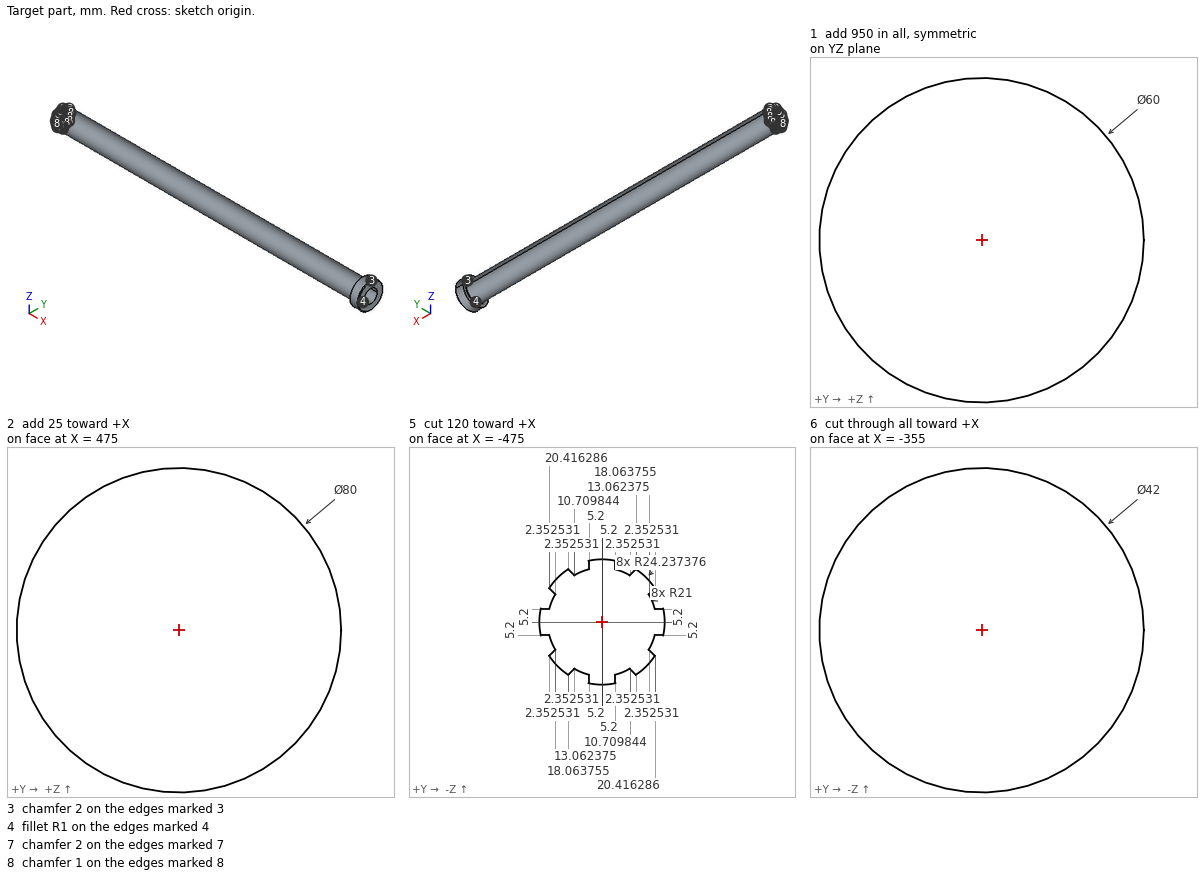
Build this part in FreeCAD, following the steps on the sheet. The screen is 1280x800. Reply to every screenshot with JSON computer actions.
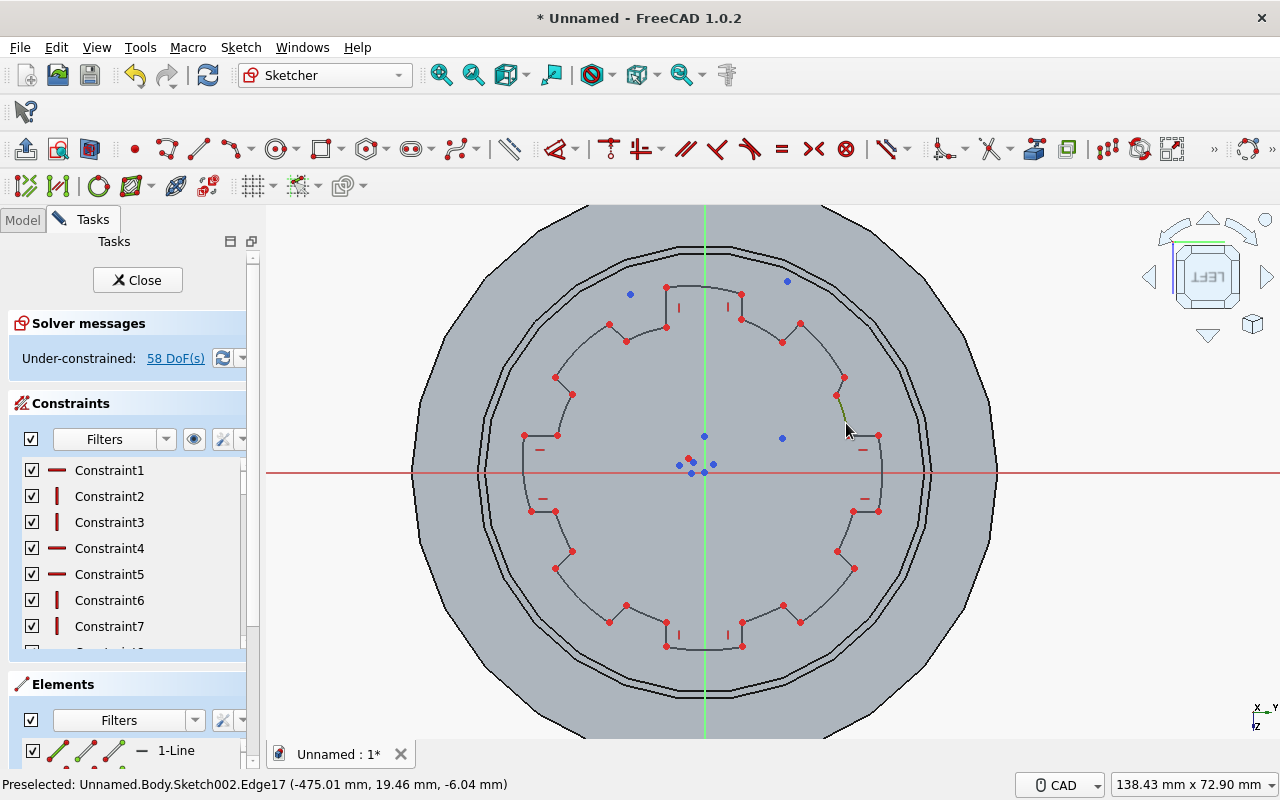
{"action": "left_click", "coordinate": [560, 524]}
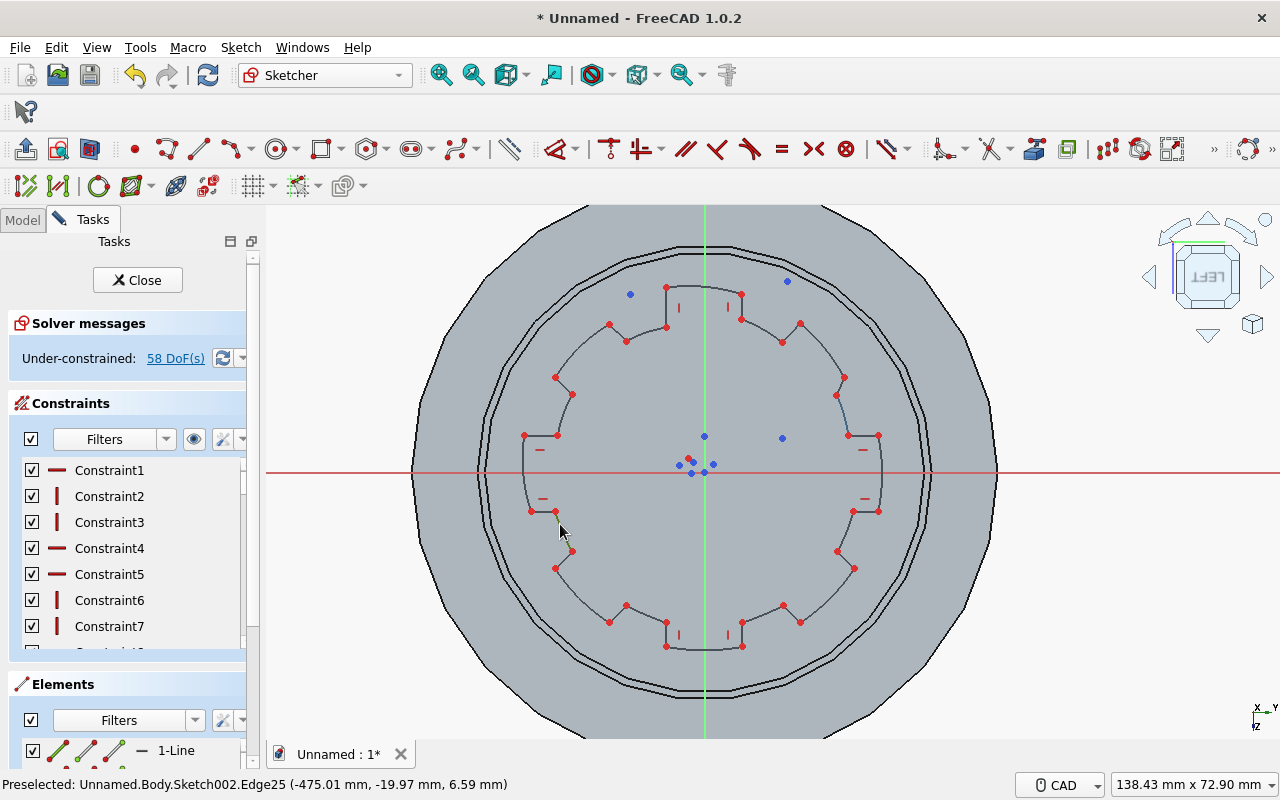
{"action": "key", "text": "c"}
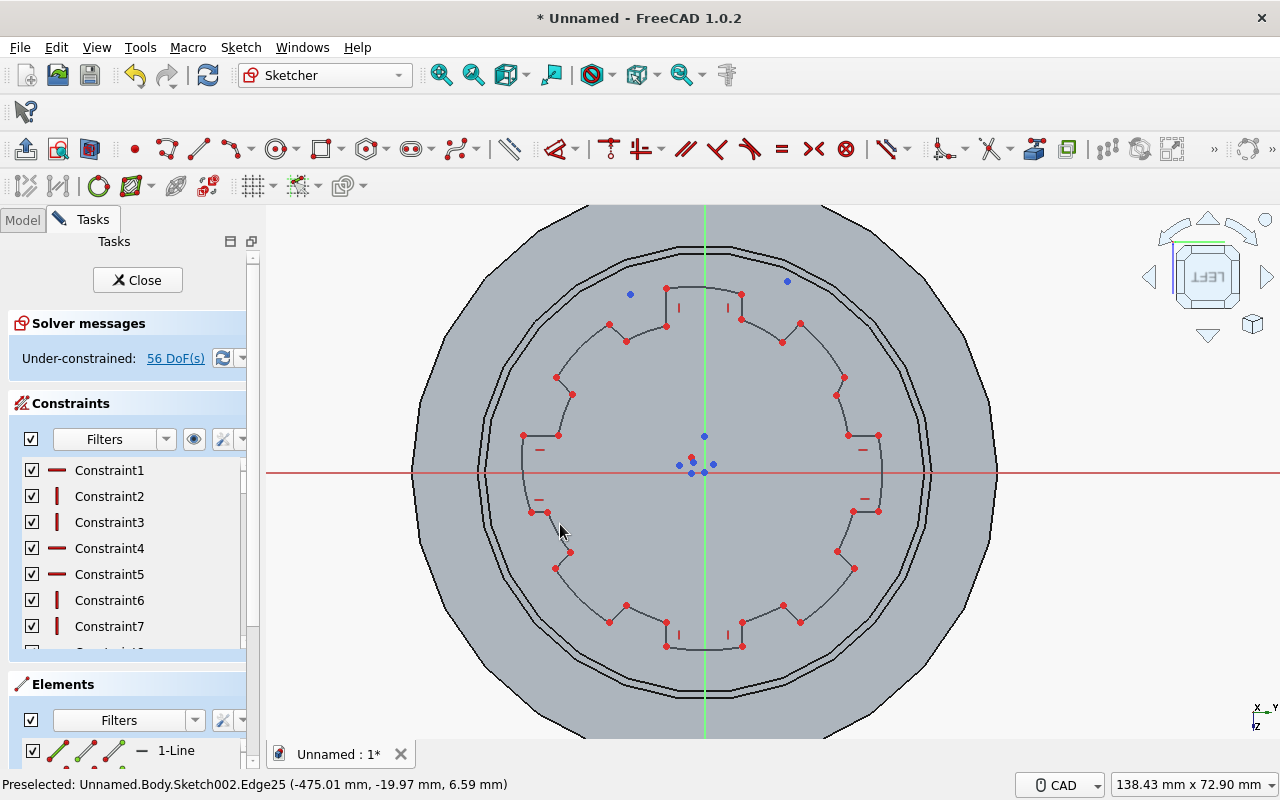
{"action": "left_click", "coordinate": [846, 423]}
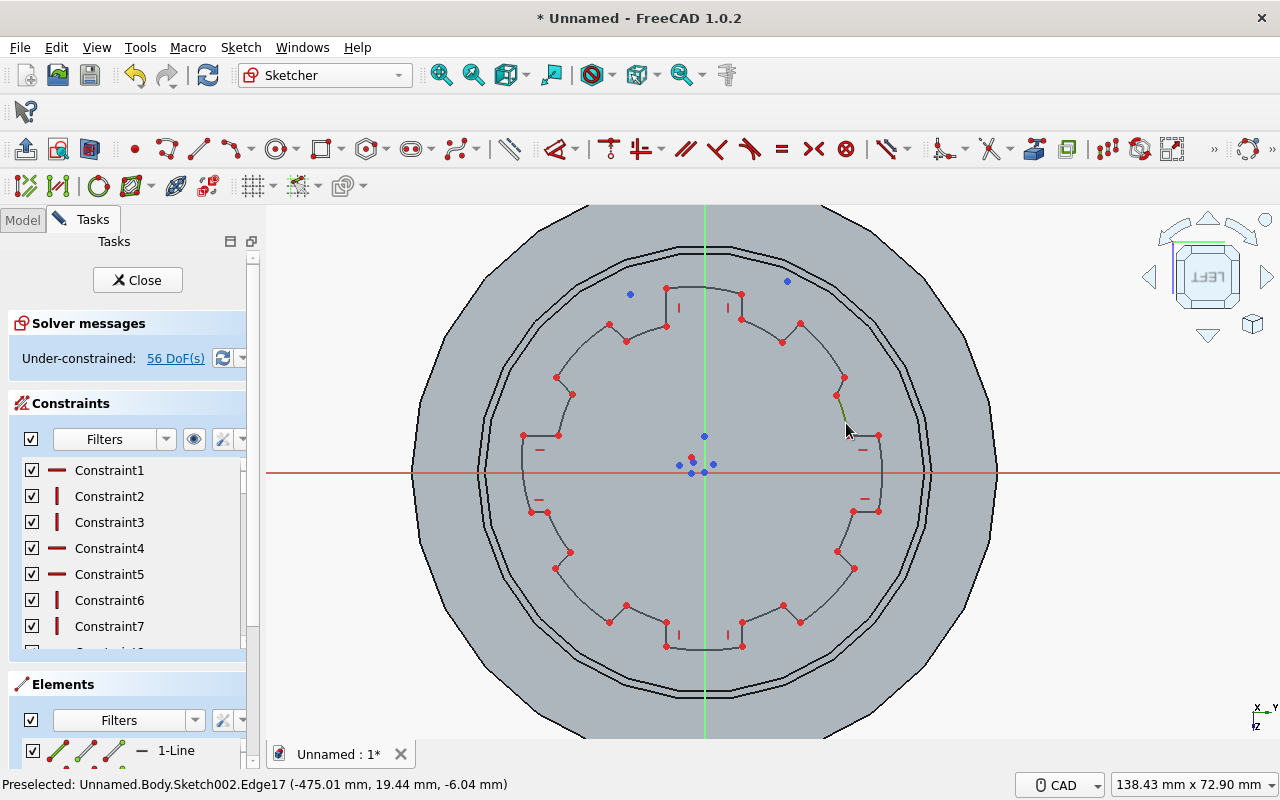
{"action": "left_click", "coordinate": [569, 587]}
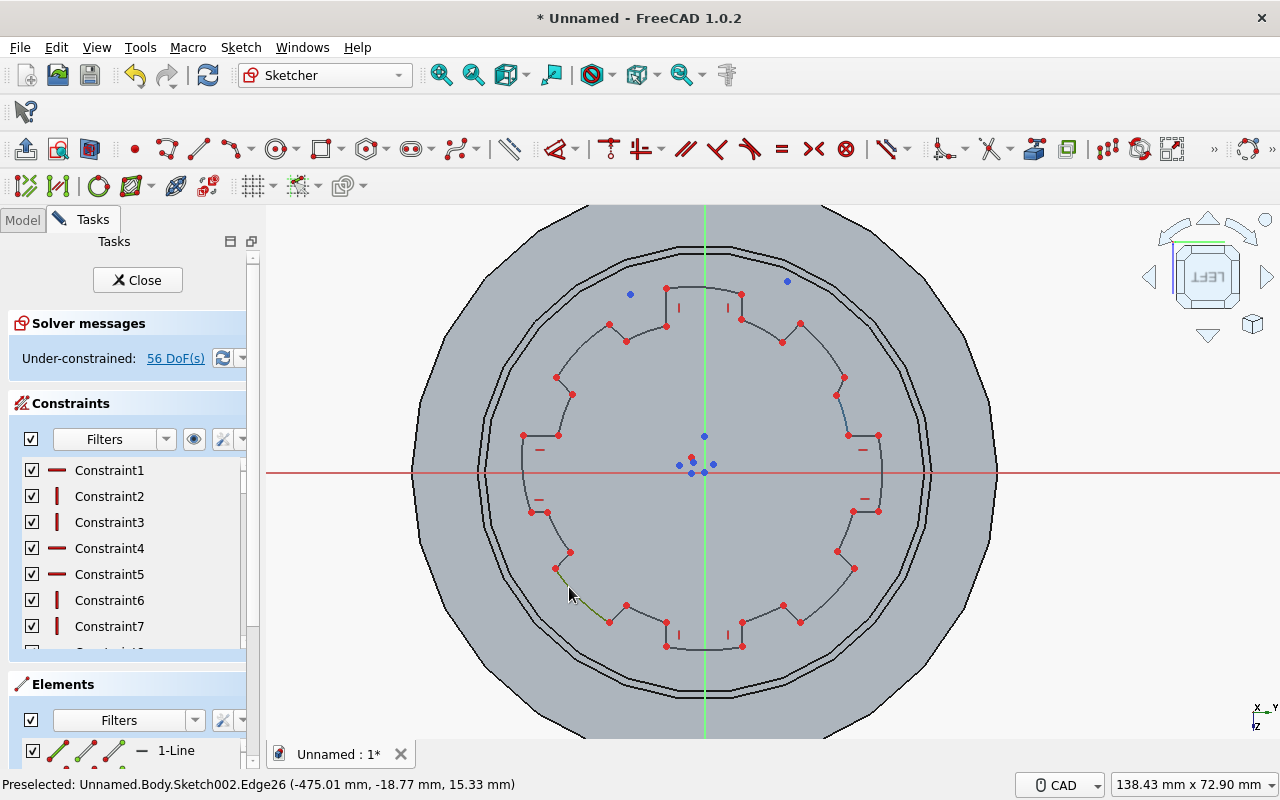
{"action": "key", "text": "c"}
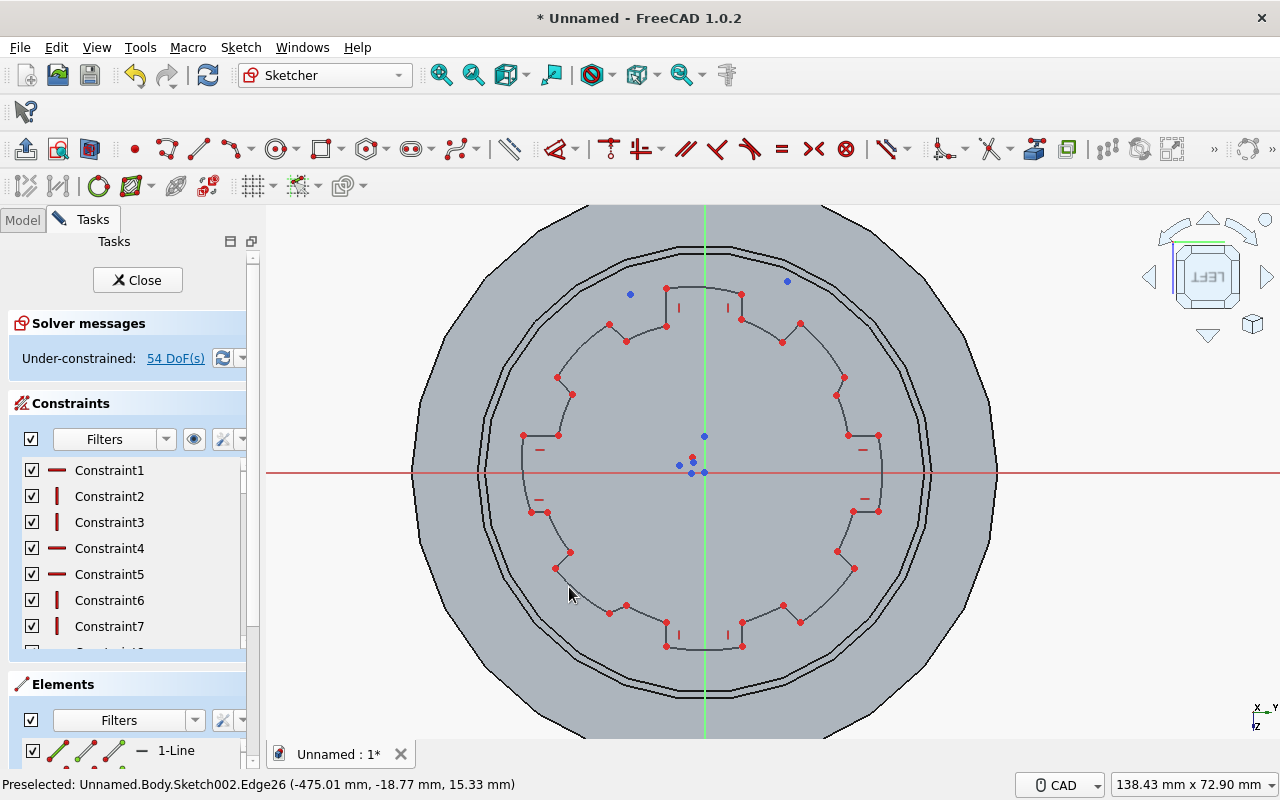
{"action": "left_click", "coordinate": [846, 423]}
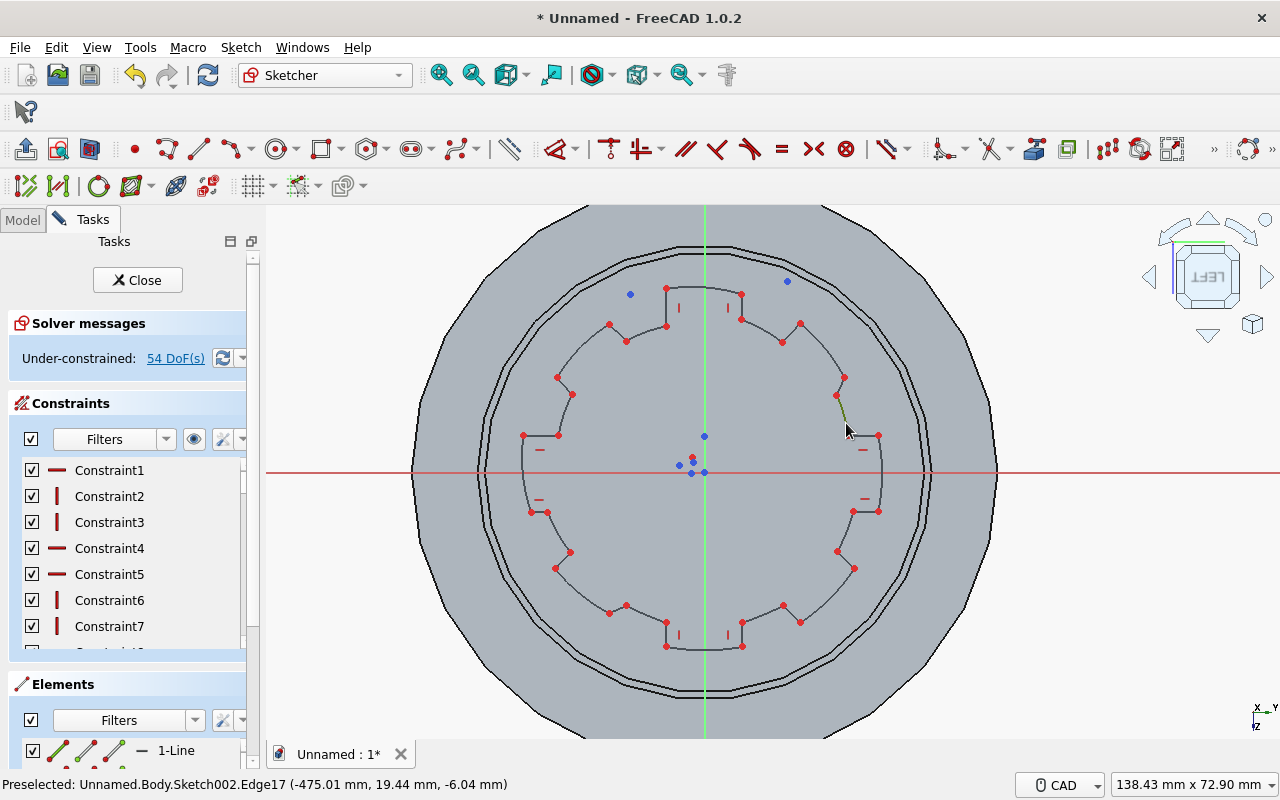
{"action": "left_click", "coordinate": [638, 611]}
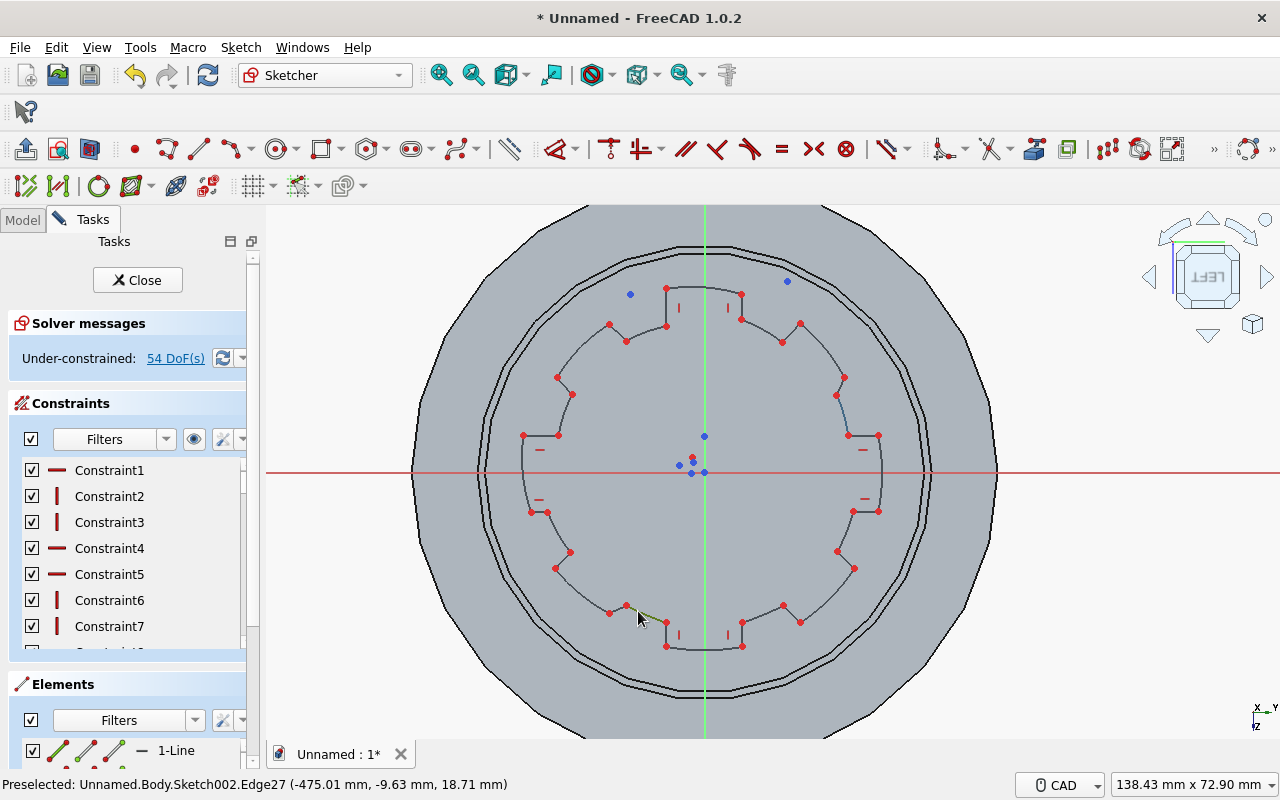
{"action": "key", "text": "c"}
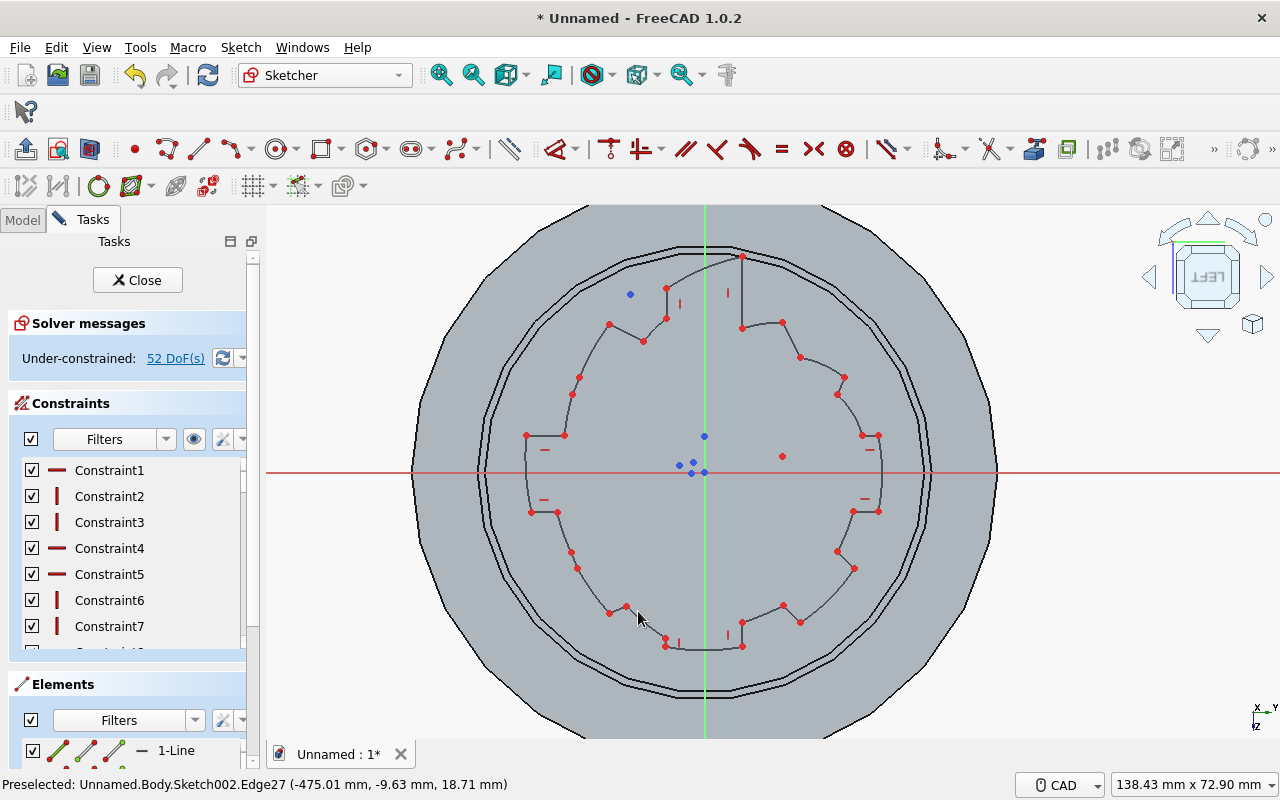
{"action": "left_click", "coordinate": [857, 422]}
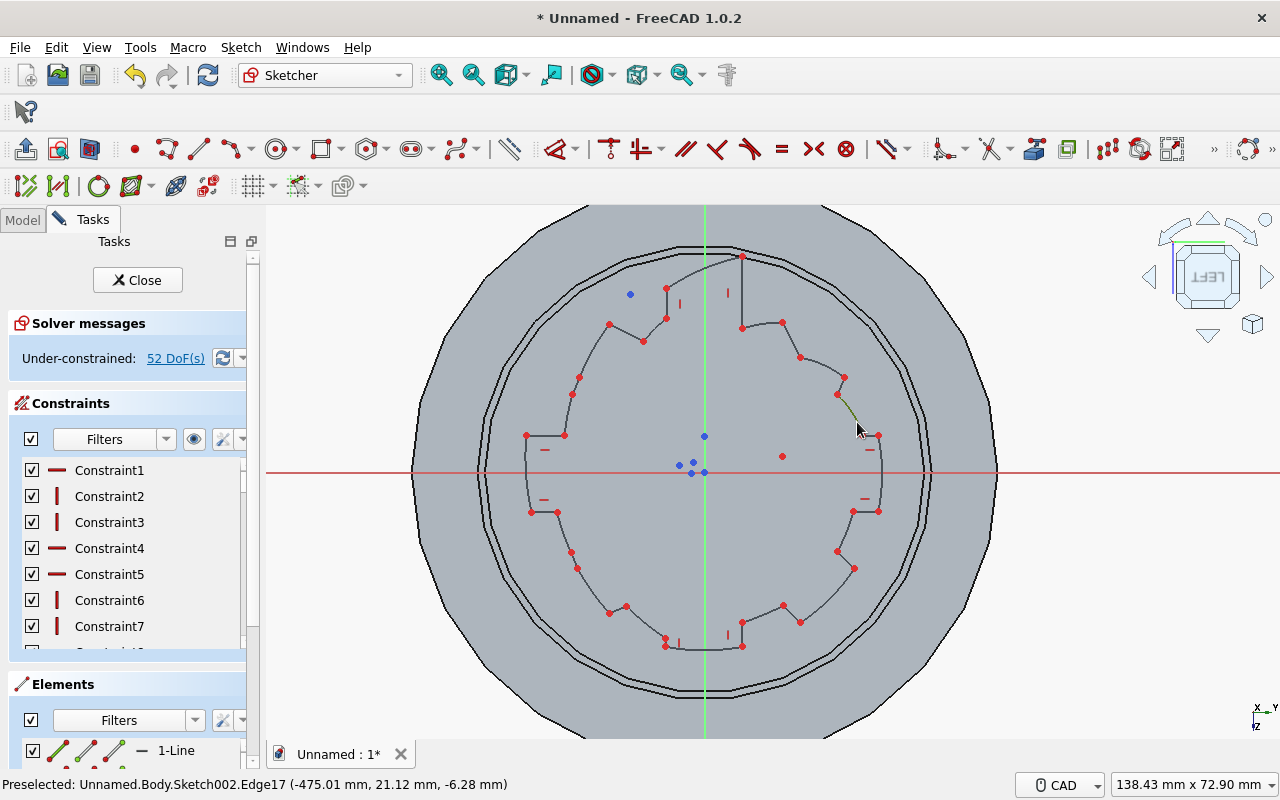
{"action": "left_click", "coordinate": [689, 650]}